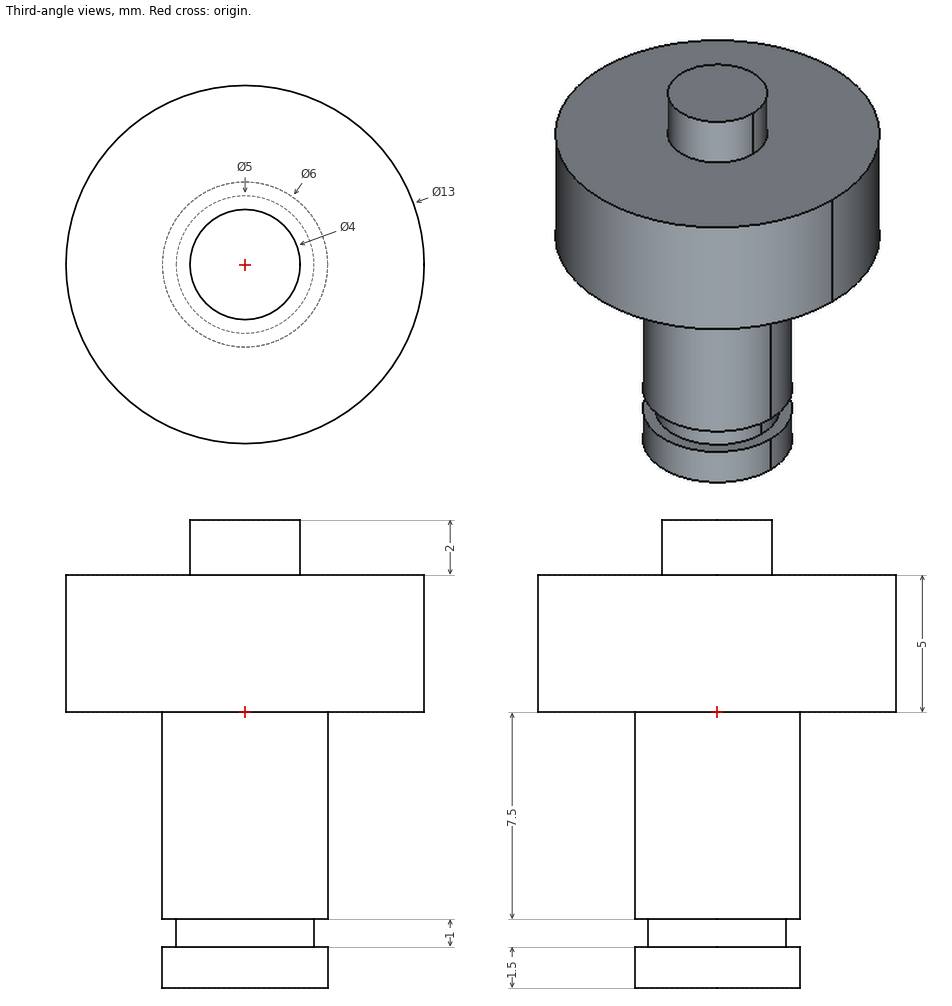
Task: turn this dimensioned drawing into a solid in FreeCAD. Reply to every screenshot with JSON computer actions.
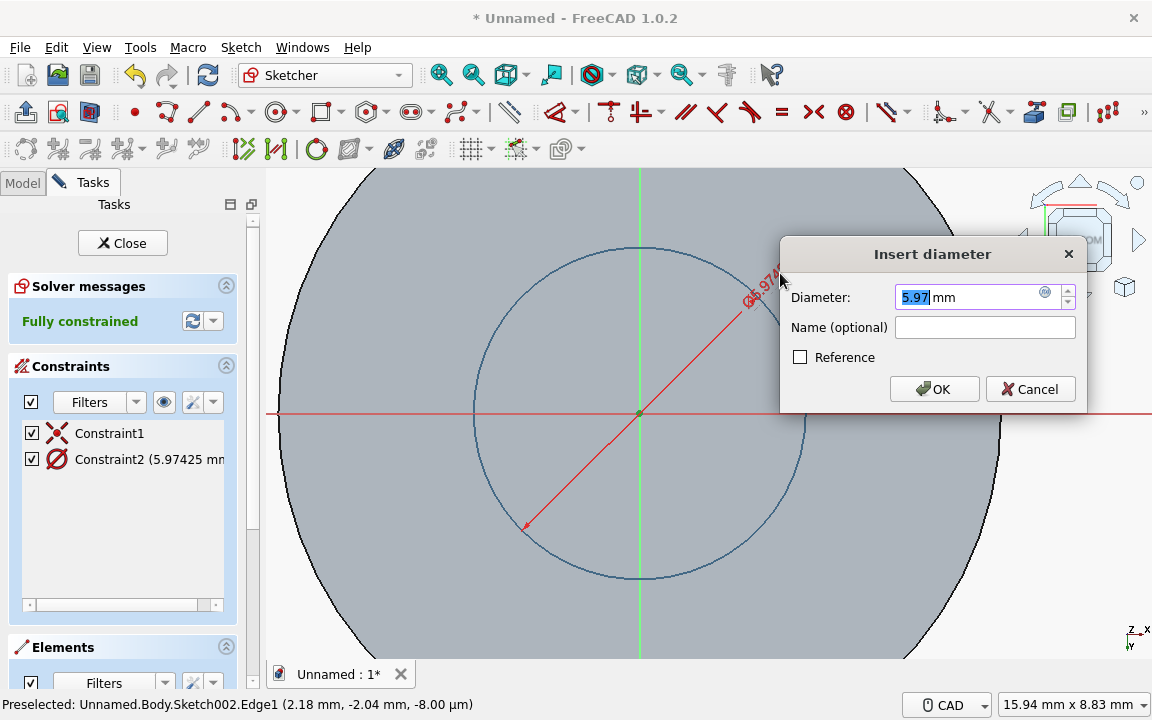
{"action": "type", "text": "6"}
{"action": "key", "text": "Return"}
{"action": "key", "text": "Escape"}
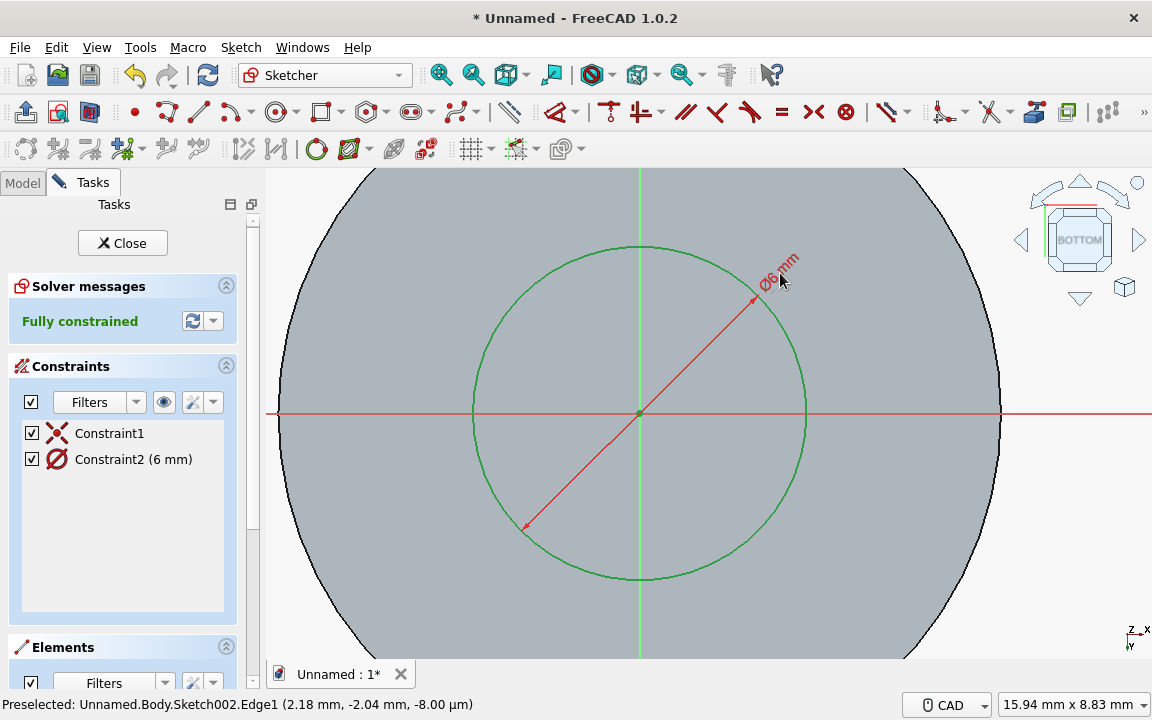
{"action": "left_click", "coordinate": [123, 243]}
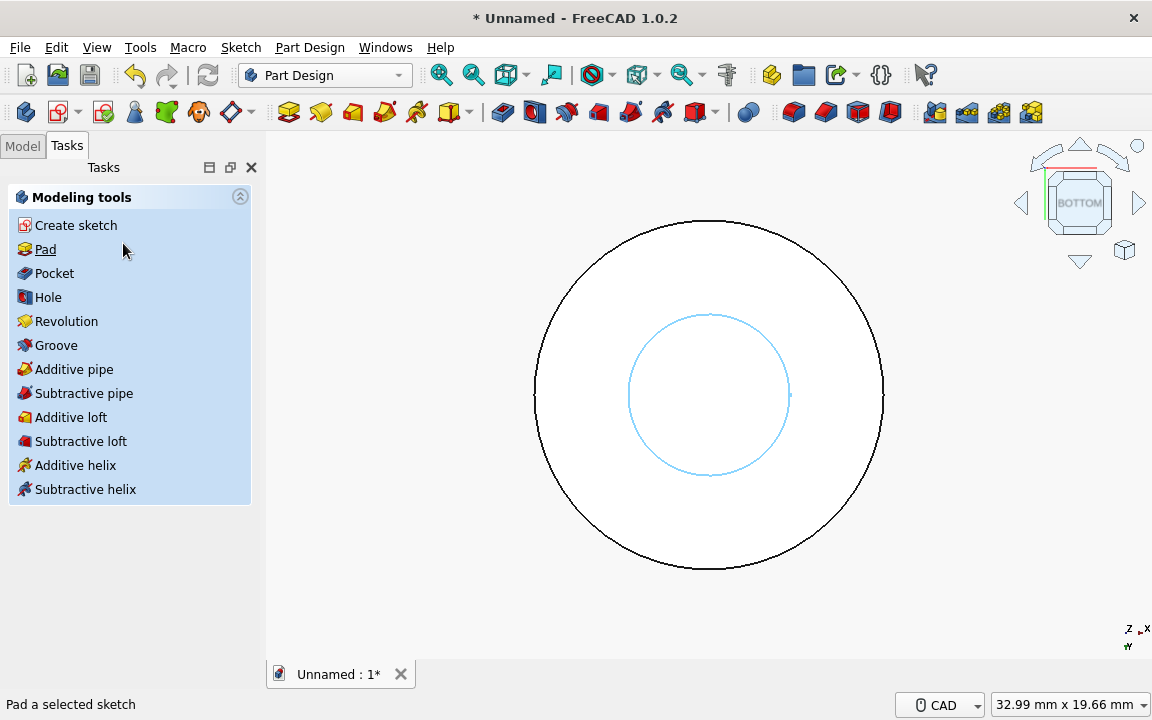
{"action": "left_click", "coordinate": [290, 112]}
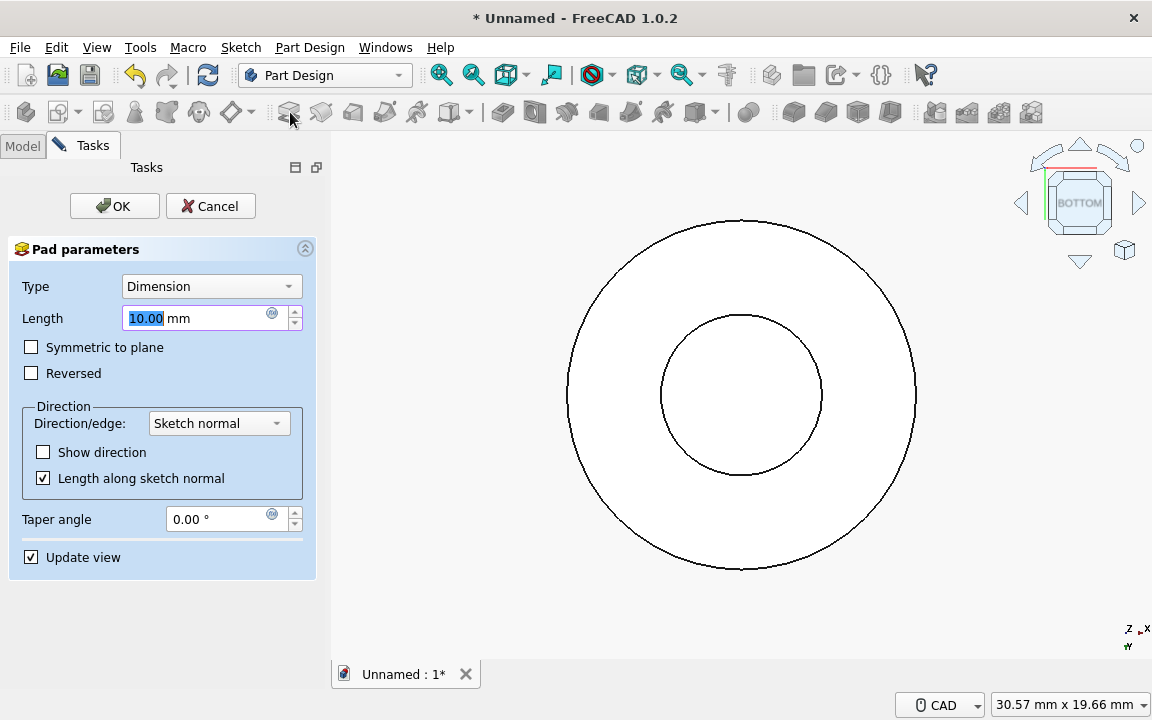
{"action": "type", "text": "7.5"}
{"action": "key", "text": "Tab"}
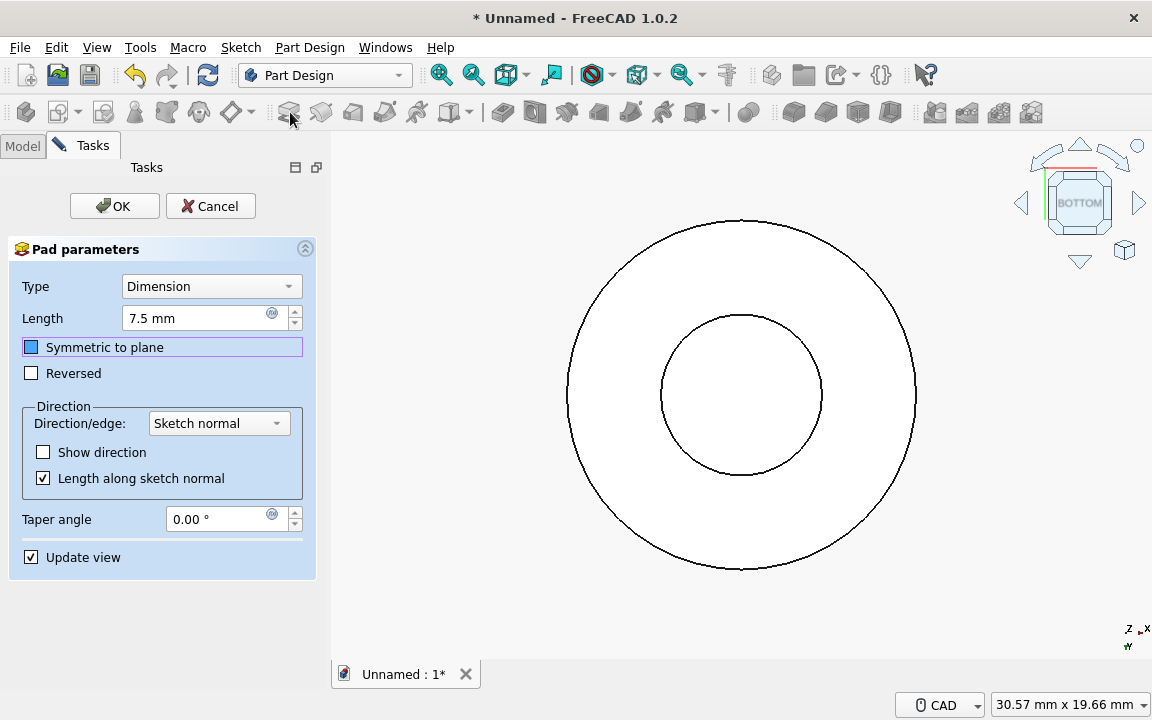
{"action": "left_click", "coordinate": [115, 206]}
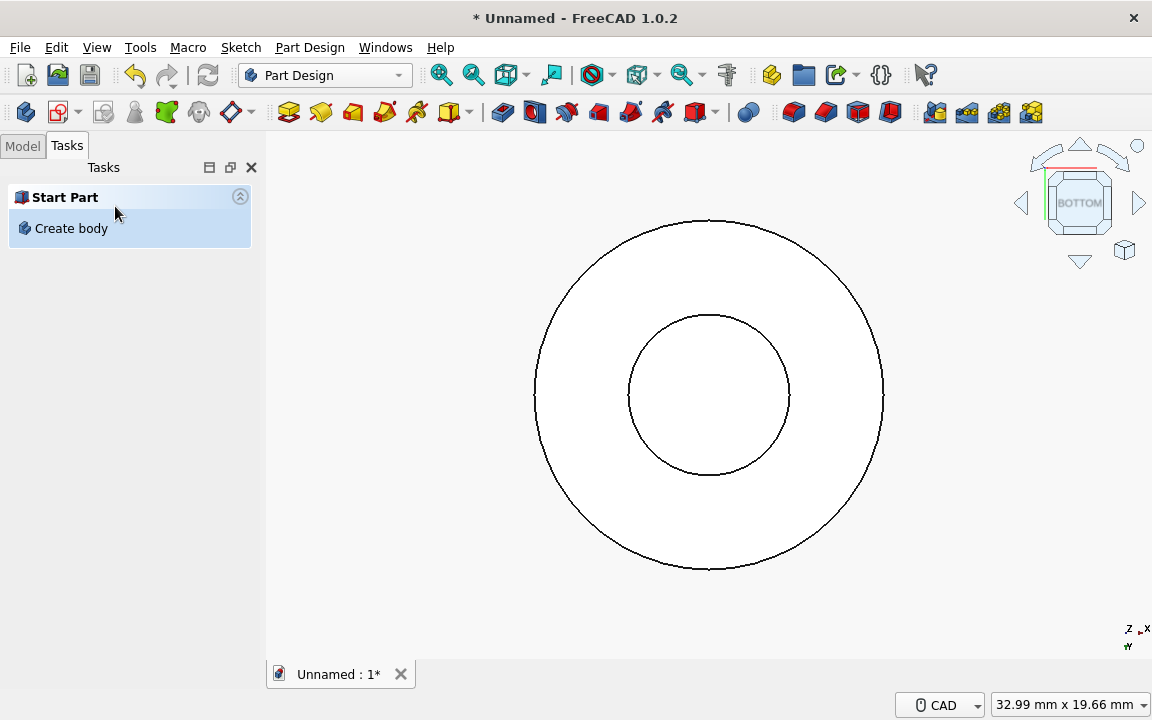
{"action": "left_click", "coordinate": [709, 394]}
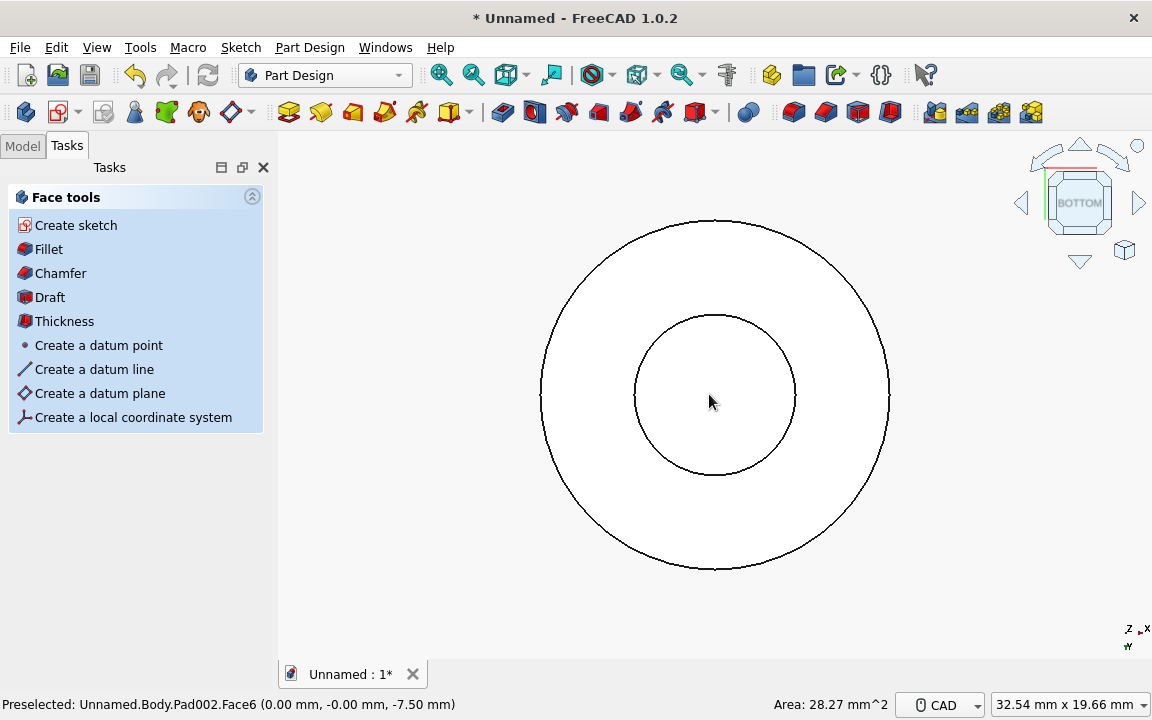
{"action": "left_click", "coordinate": [58, 112]}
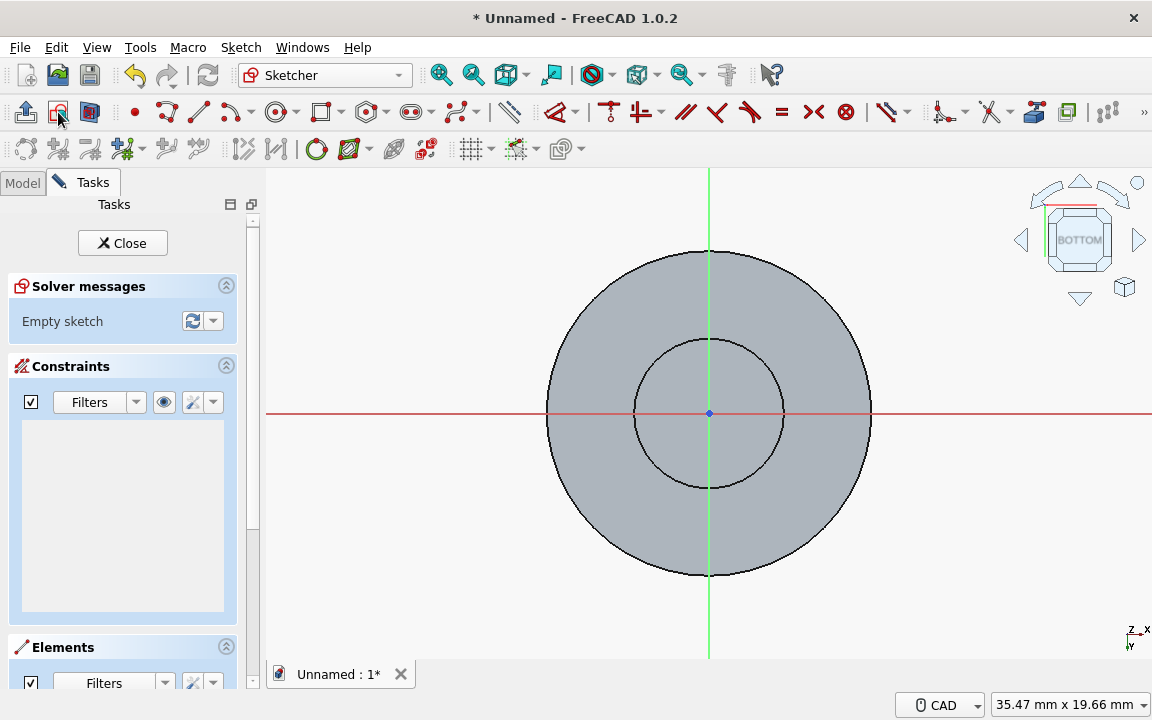
{"action": "scroll", "coordinate": [765, 414], "scroll_direction": "up", "scroll_amount": 4}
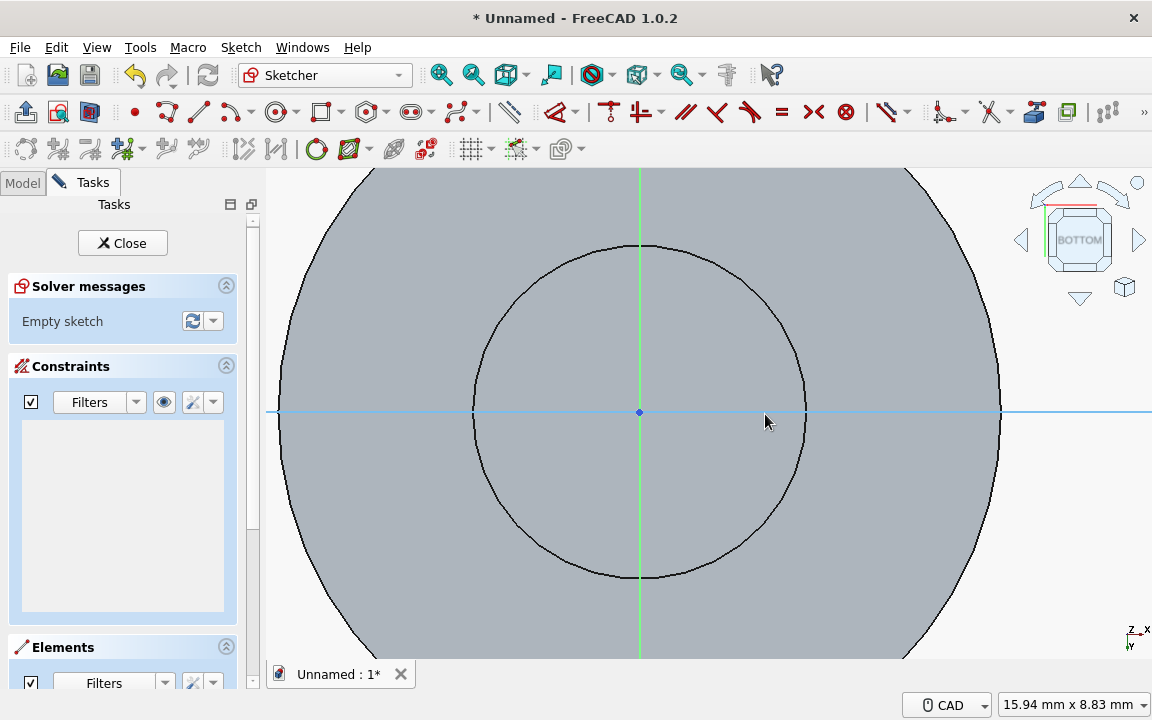
{"action": "key", "text": "g c"}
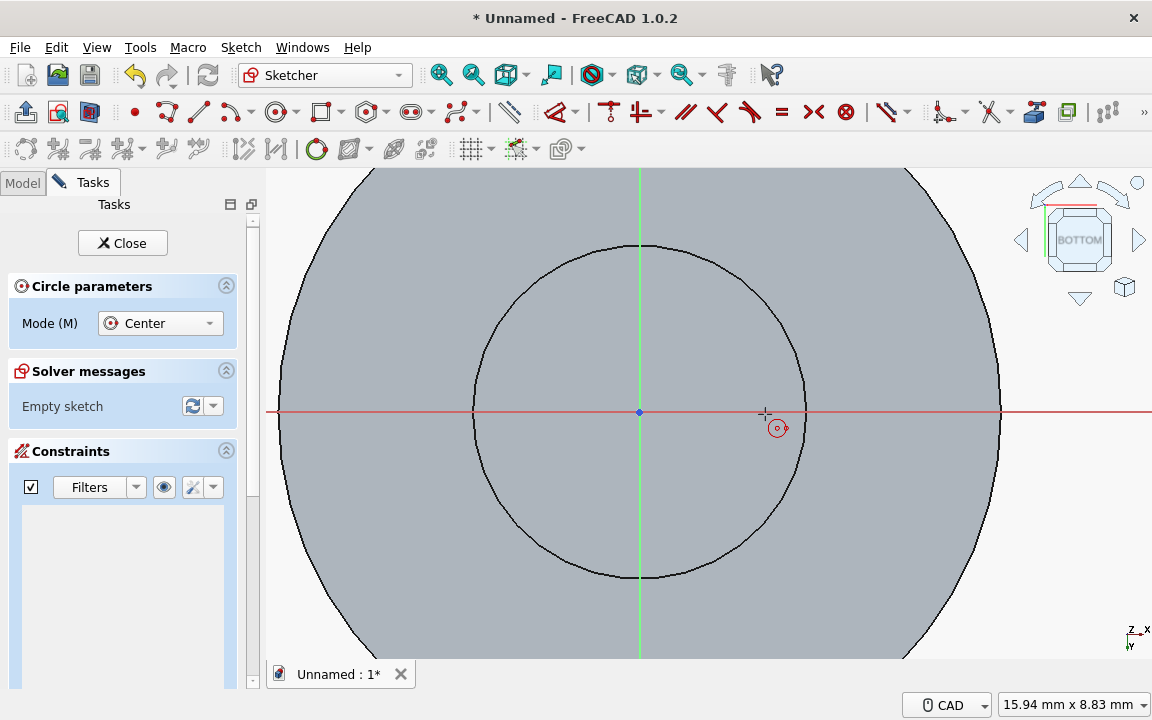
{"action": "left_click", "coordinate": [640, 412]}
{"action": "left_click", "coordinate": [738, 314]}
{"action": "key", "text": "Escape"}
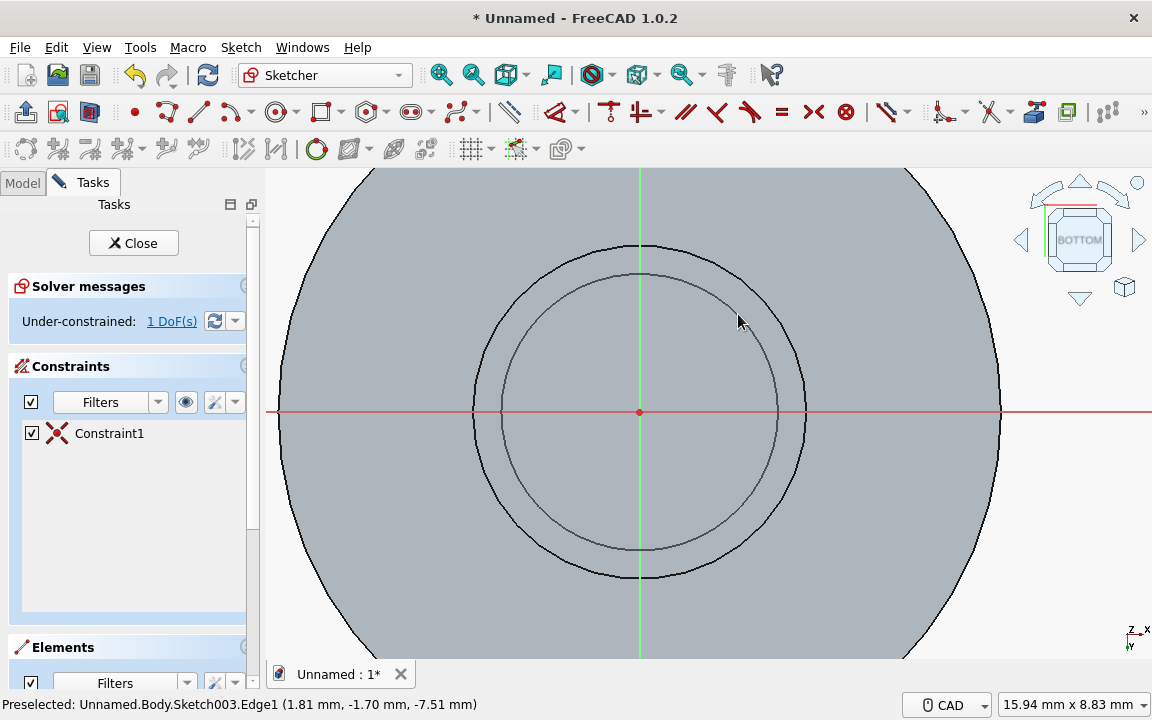
{"action": "key", "text": "d"}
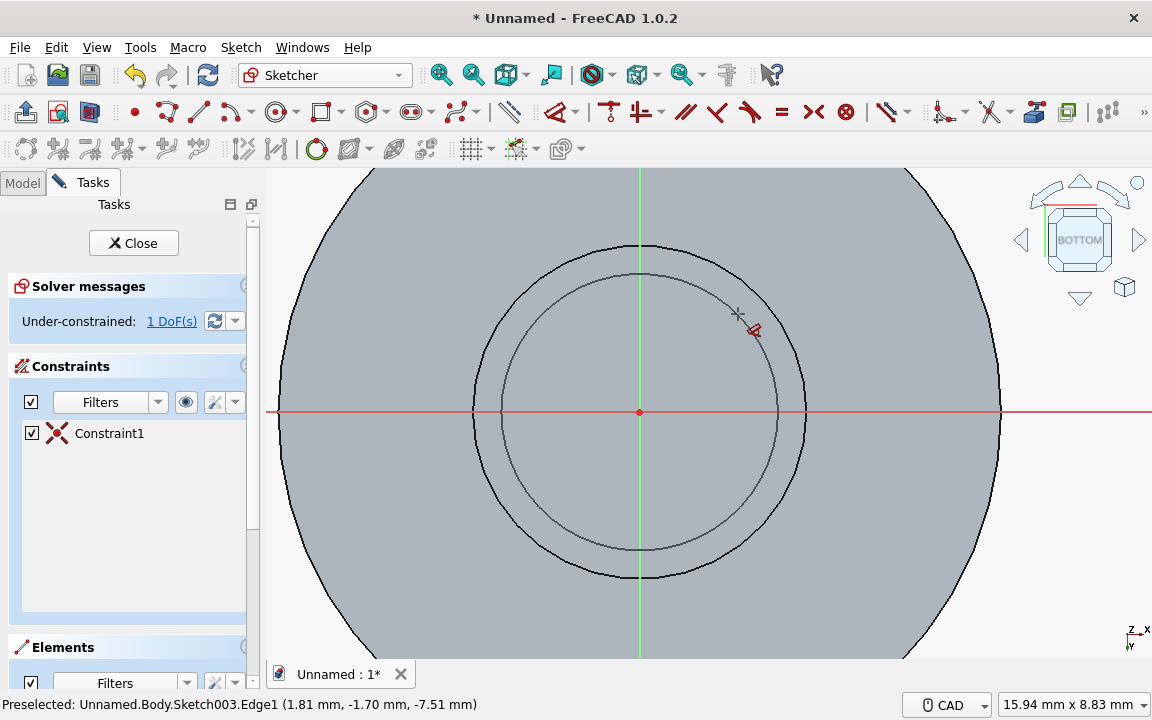
{"action": "left_click", "coordinate": [737, 314]}
{"action": "left_click", "coordinate": [760, 291]}